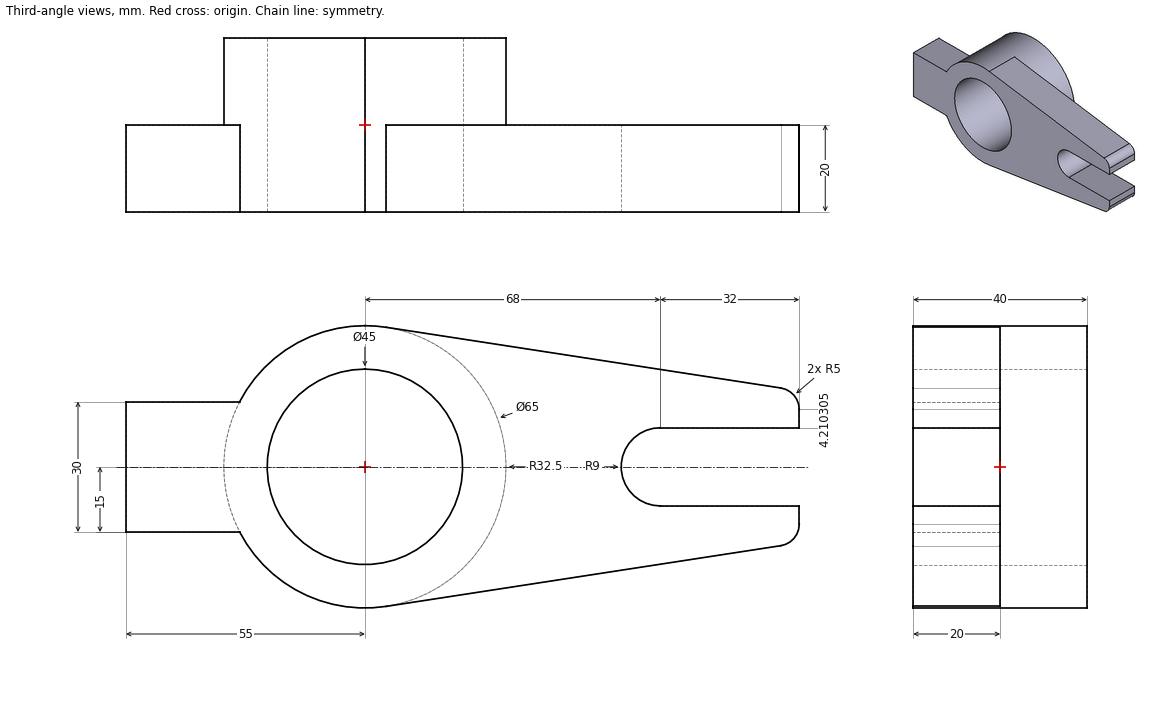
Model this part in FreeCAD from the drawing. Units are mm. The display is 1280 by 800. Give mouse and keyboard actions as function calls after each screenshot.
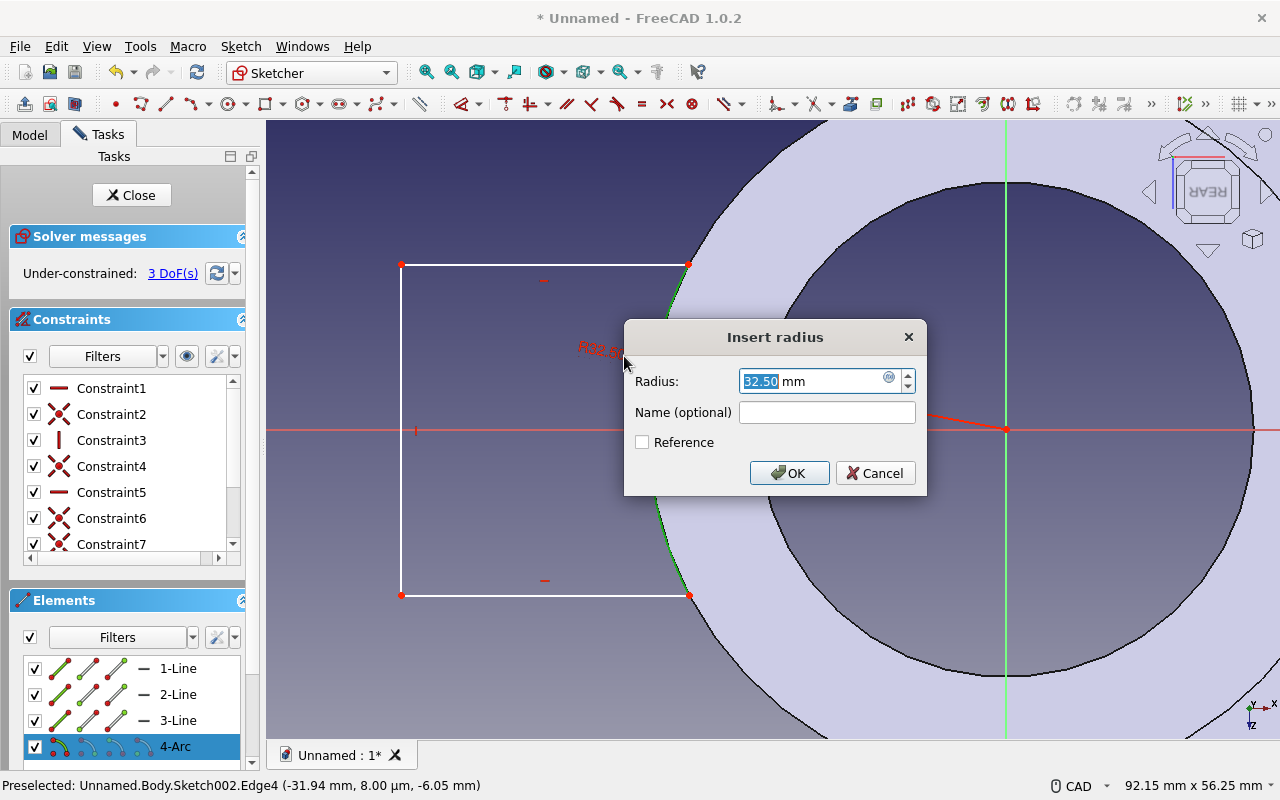
text(32.5)
key(Return)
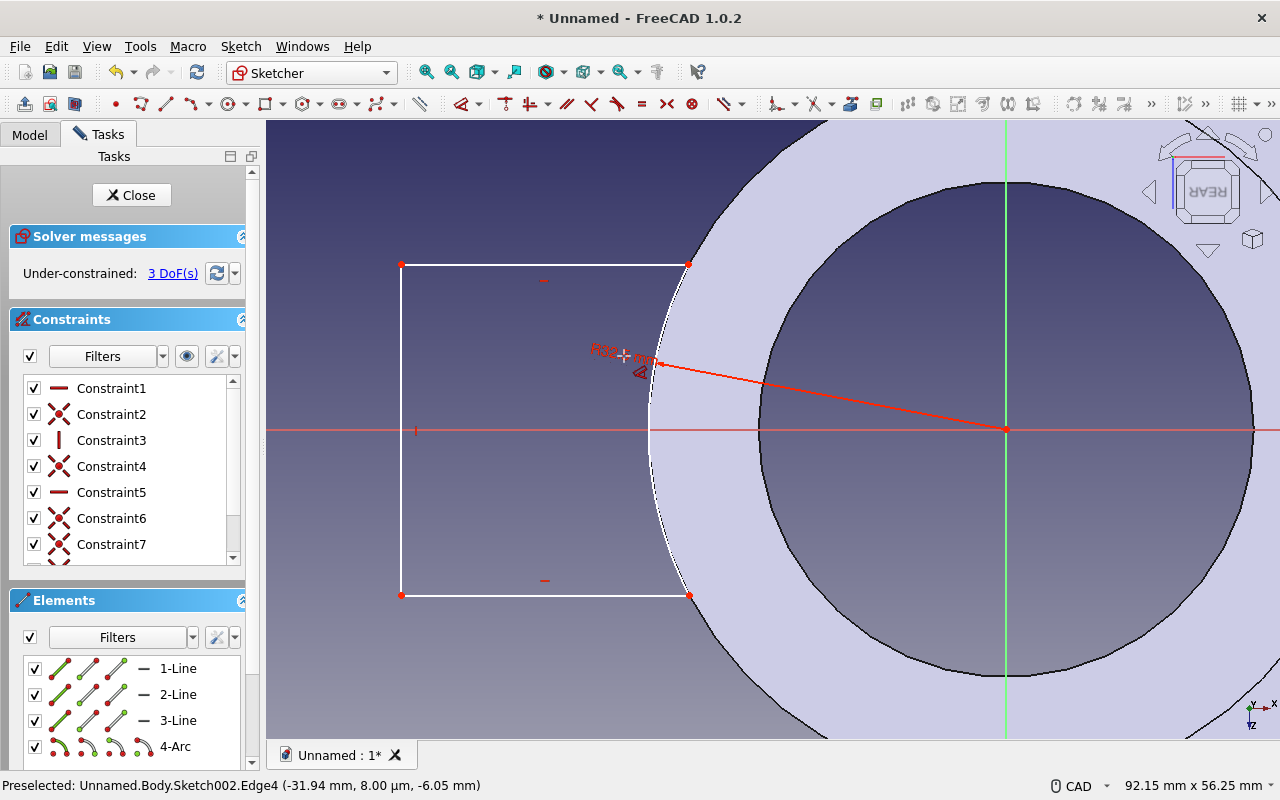
click(401, 364)
click(367, 354)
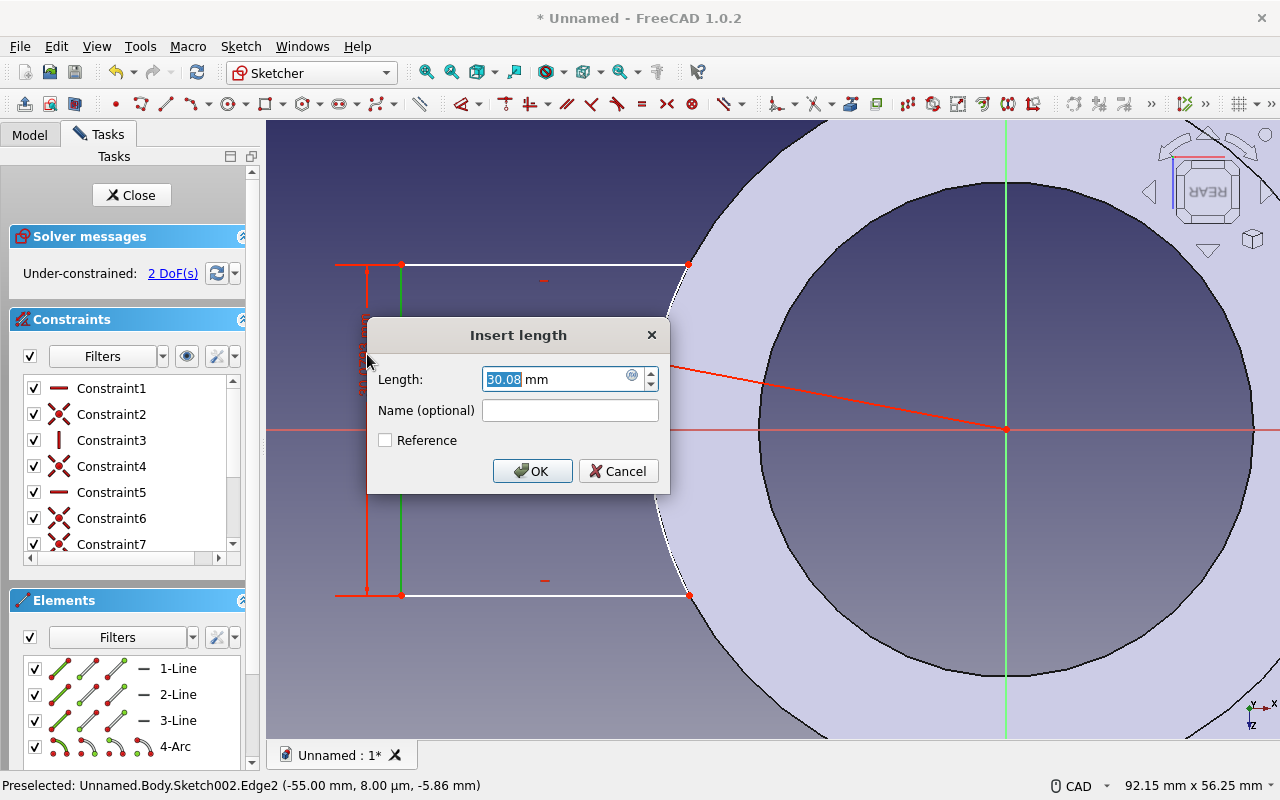
text(30)
key(Return)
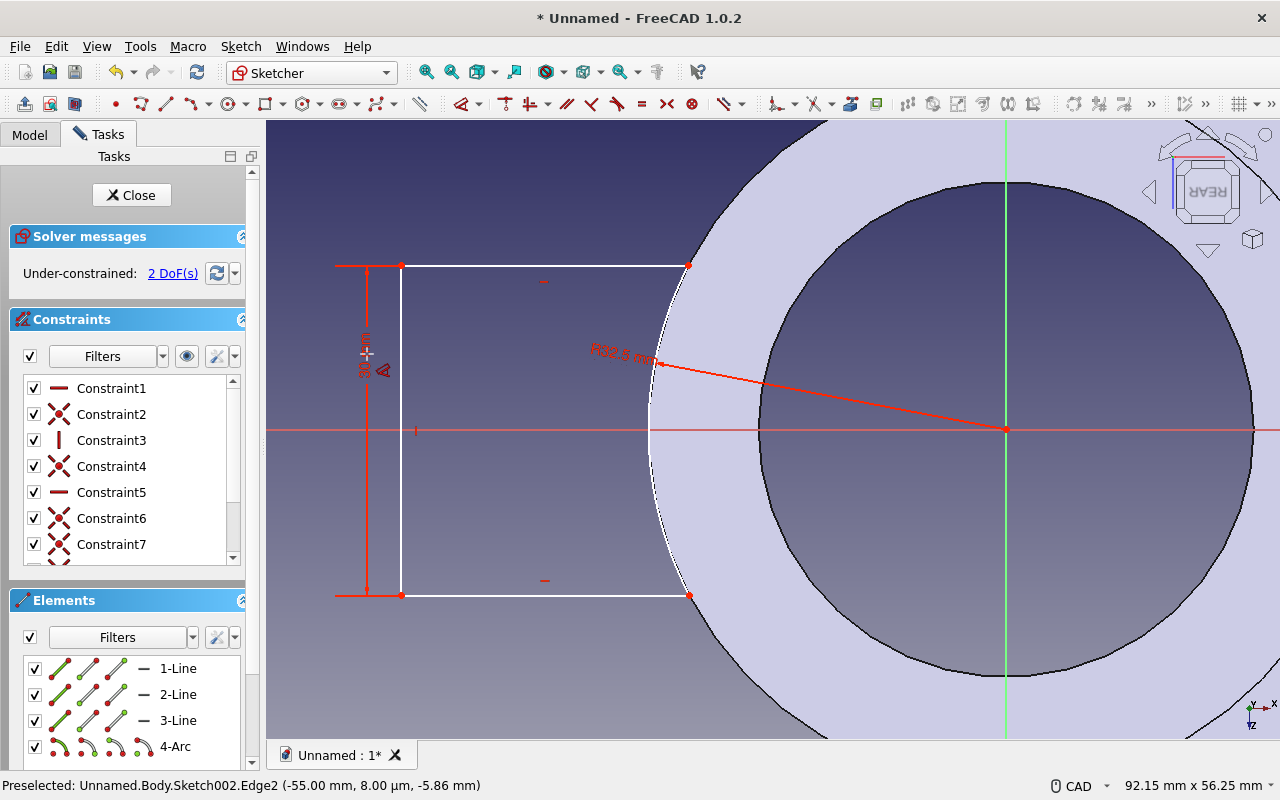
click(688, 266)
click(1040, 348)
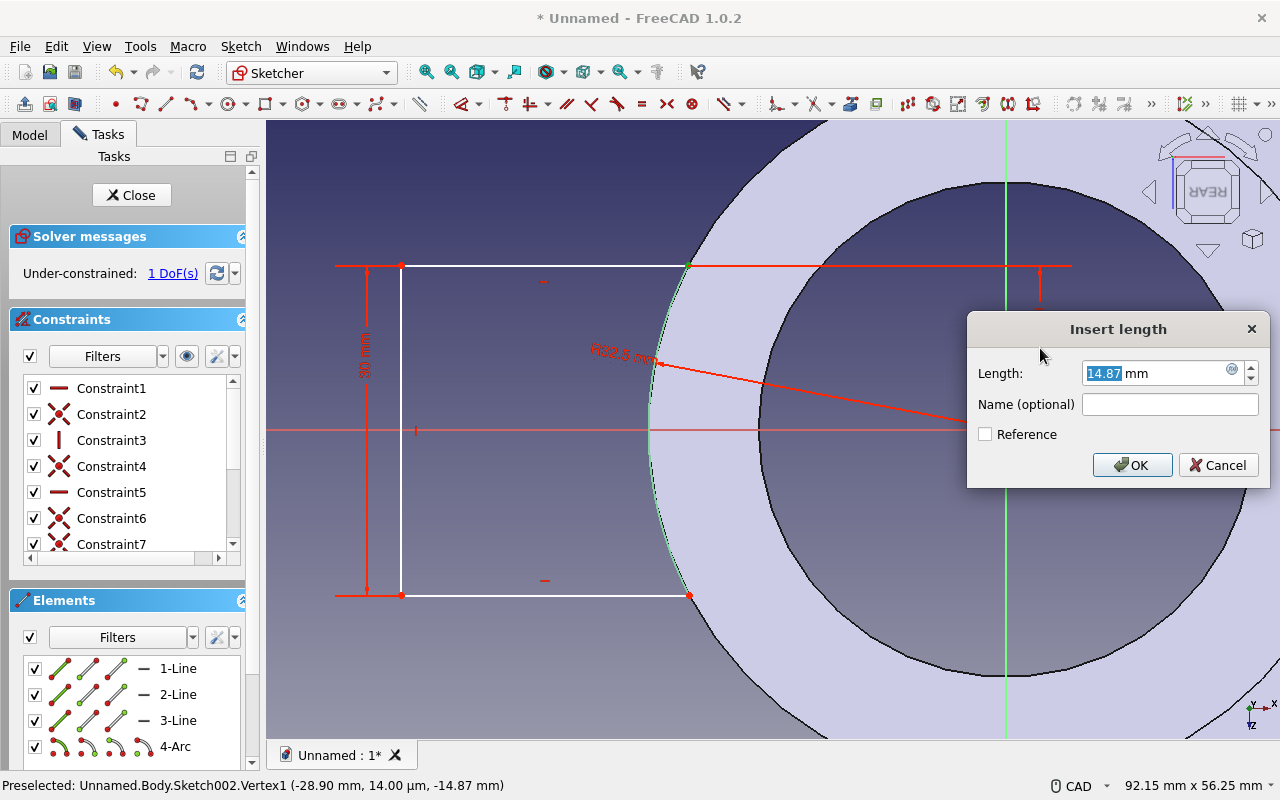
text(15)
key(Return)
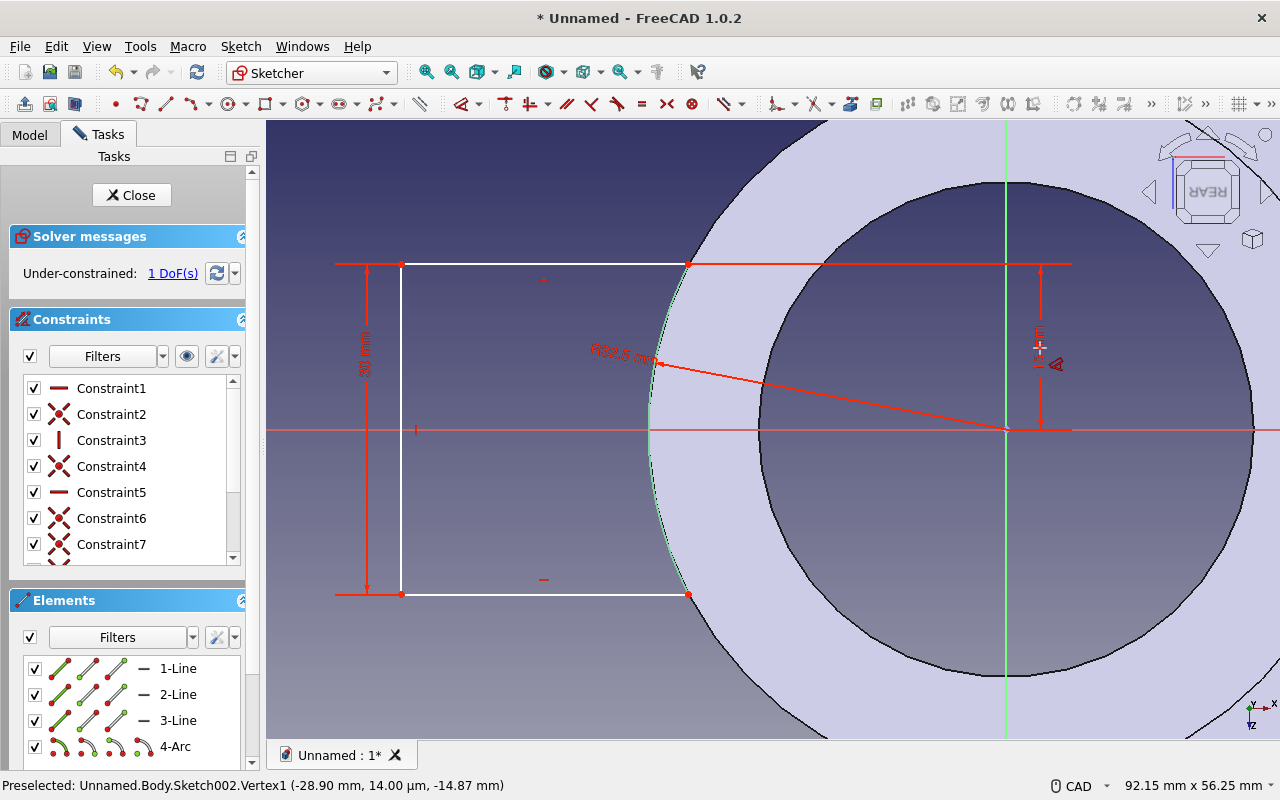
click(401, 264)
click(704, 230)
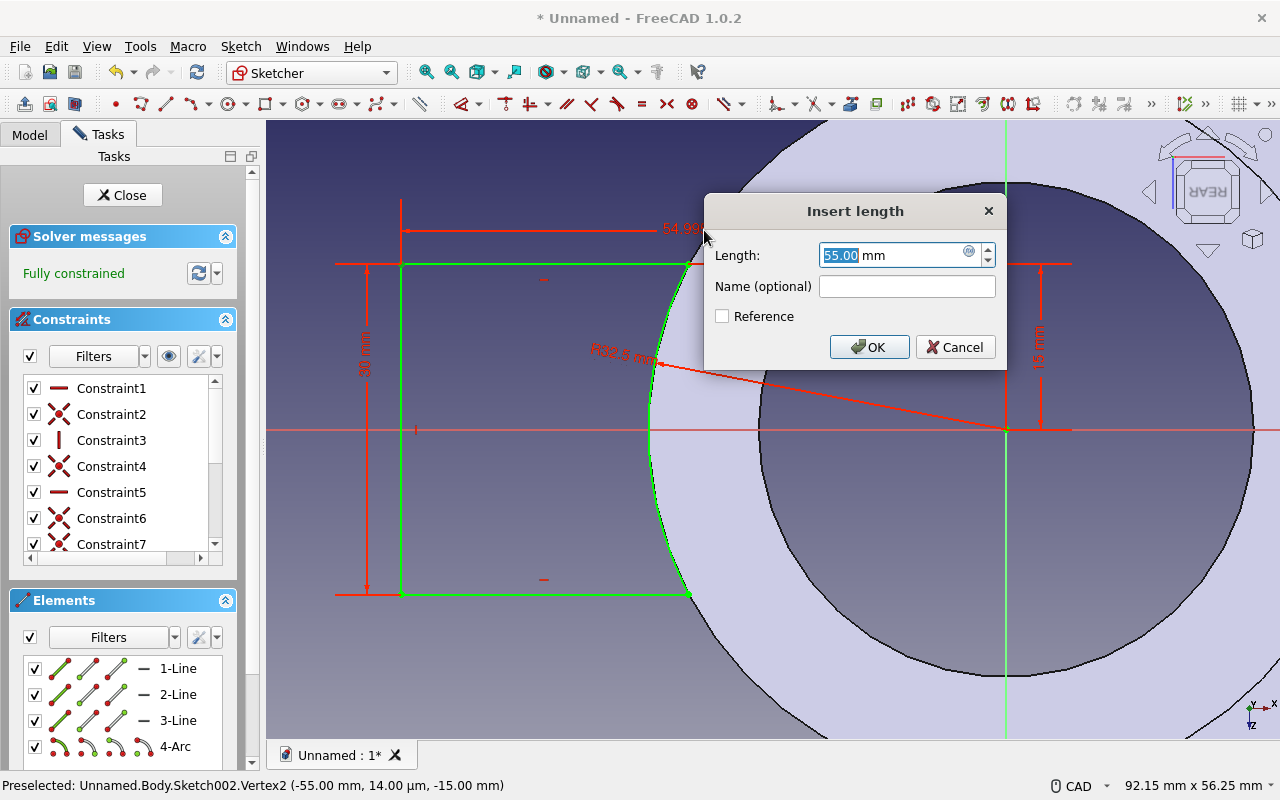
text(55)
key(Return)
key(Escape)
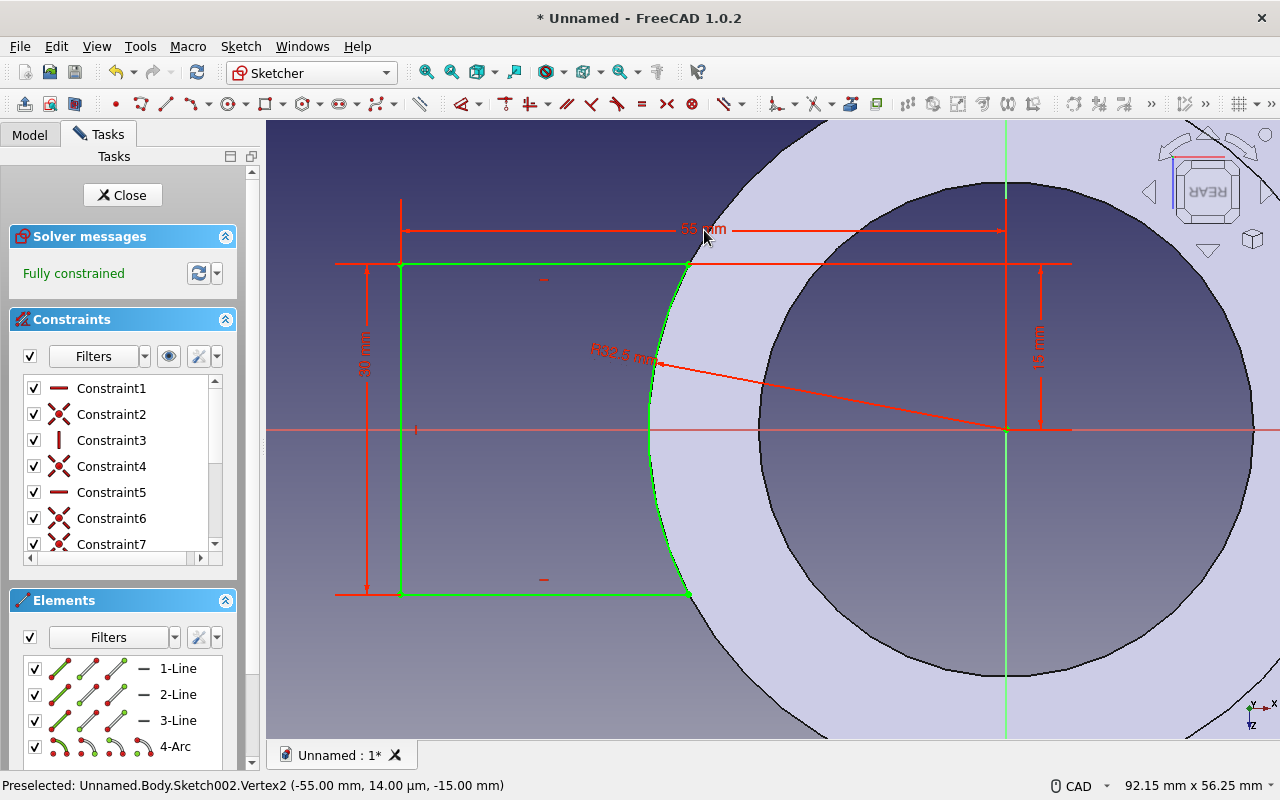
click(123, 195)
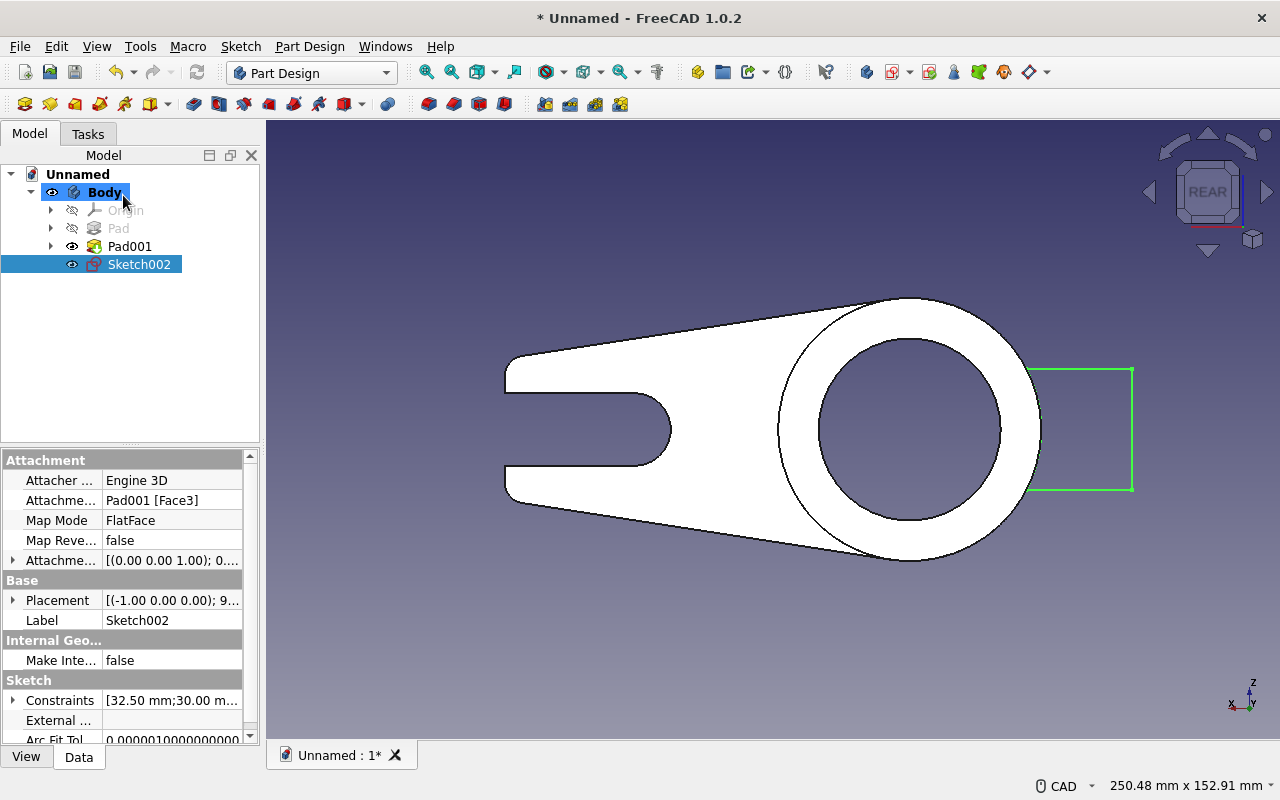
click(25, 104)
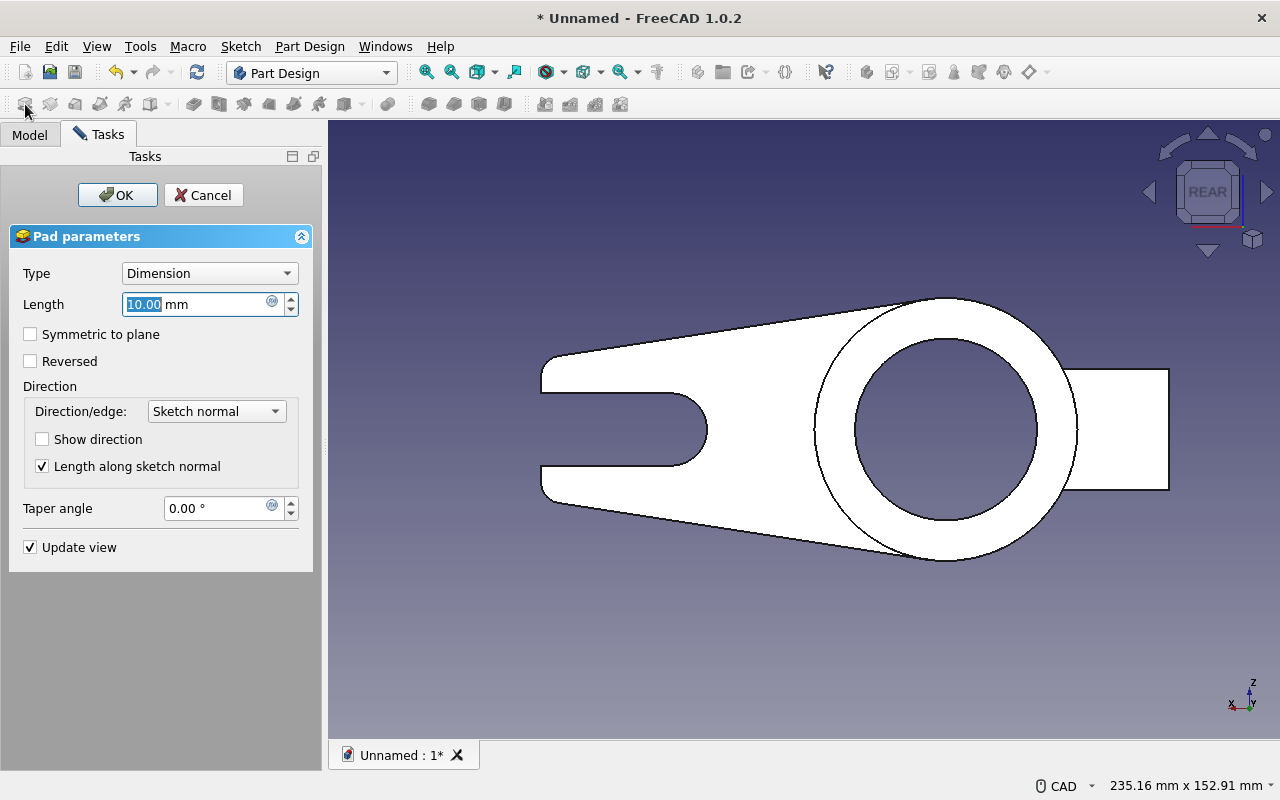
text(20)
key(Tab)